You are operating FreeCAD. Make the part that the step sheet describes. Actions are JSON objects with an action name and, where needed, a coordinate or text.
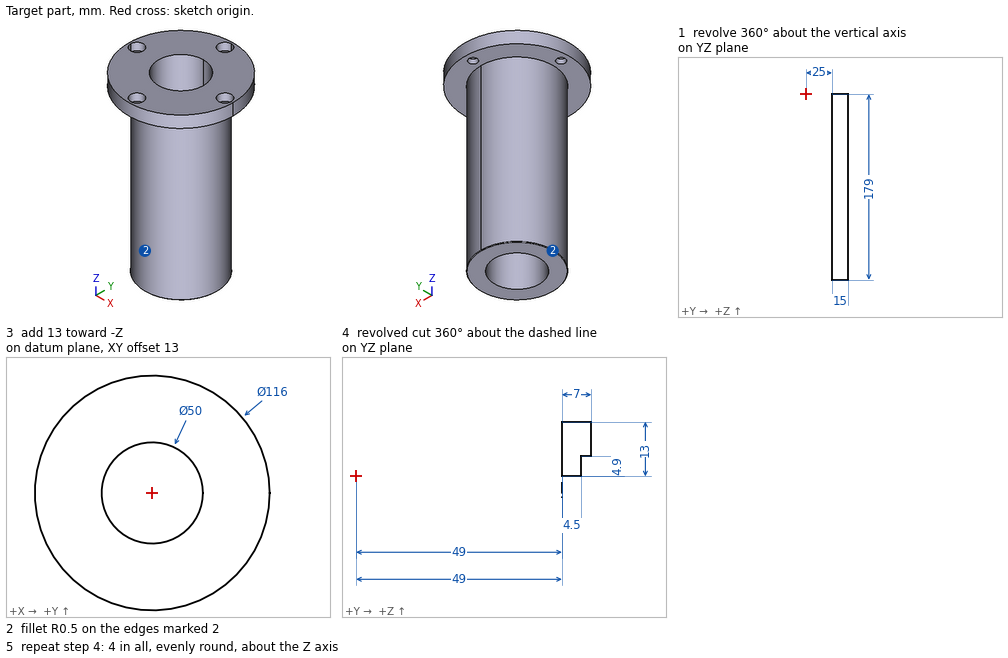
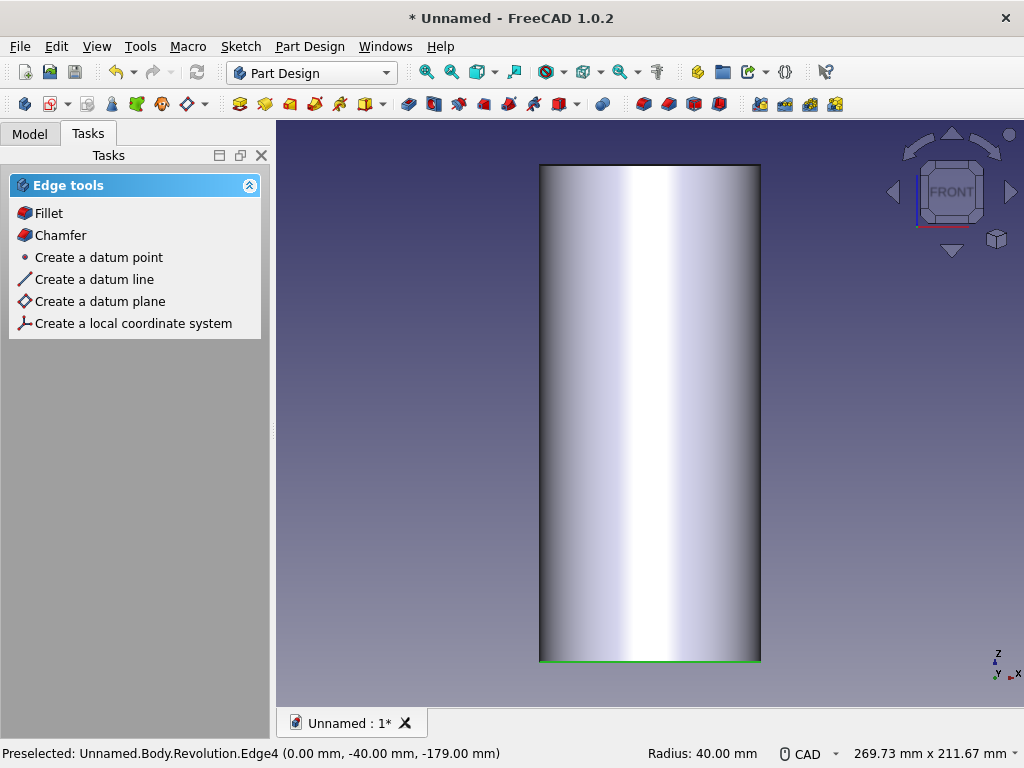
{"action": "left_click", "coordinate": [644, 104]}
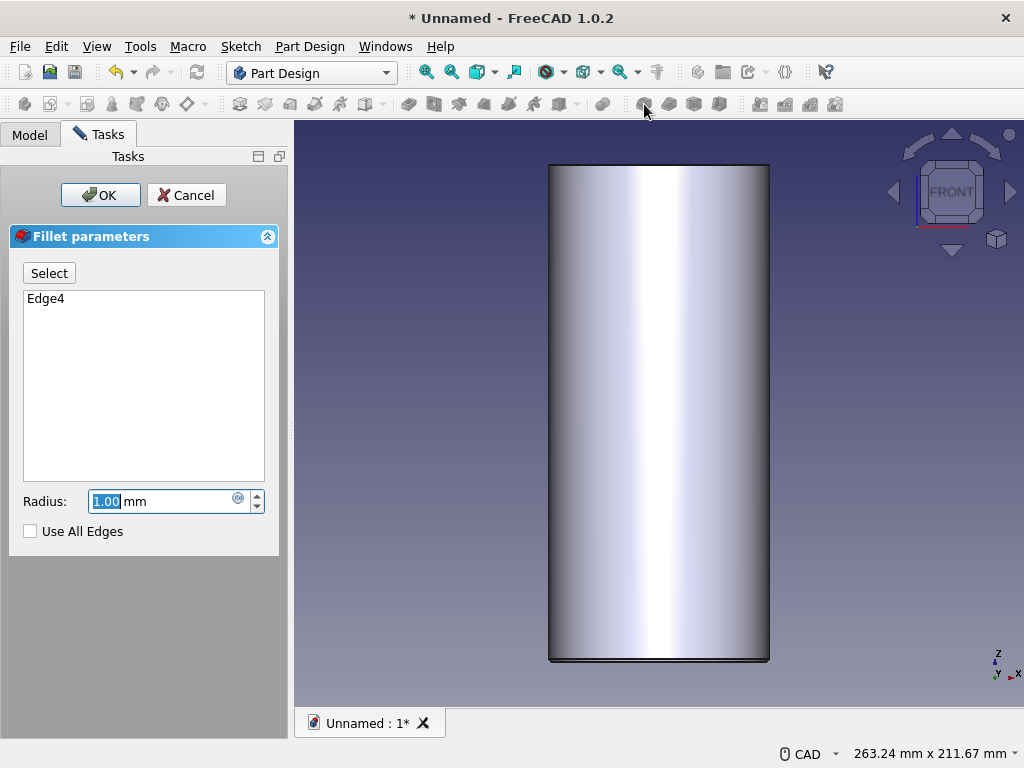
{"action": "type", "text": "0.5"}
{"action": "key", "text": "Tab"}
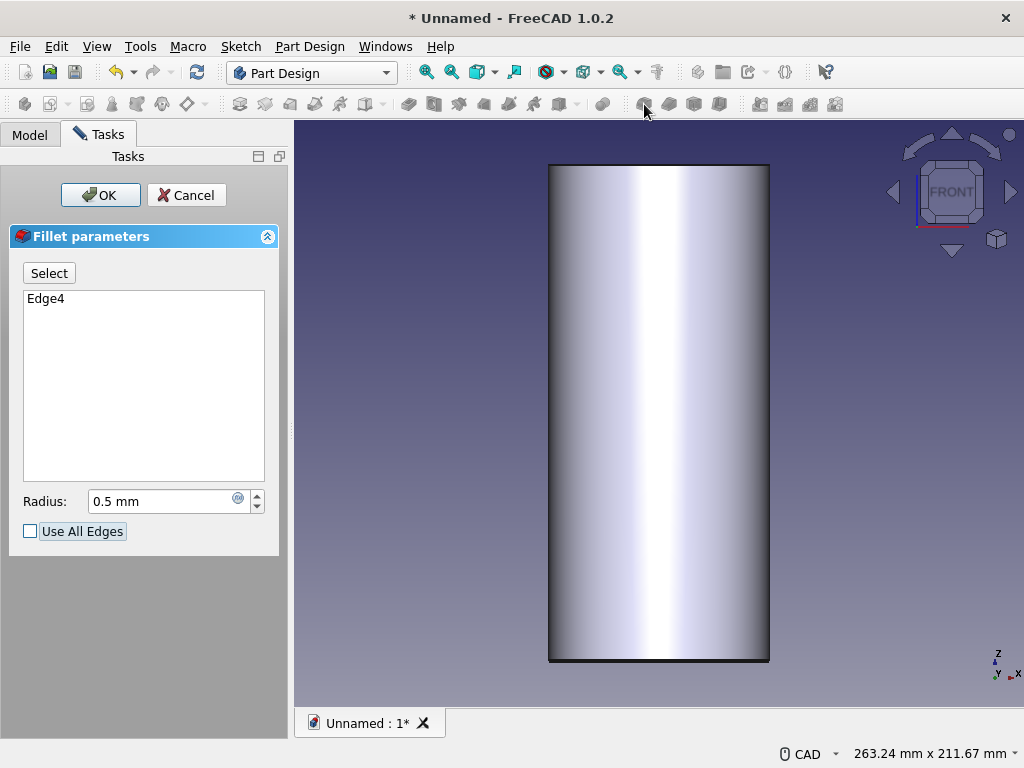
{"action": "left_click", "coordinate": [101, 195]}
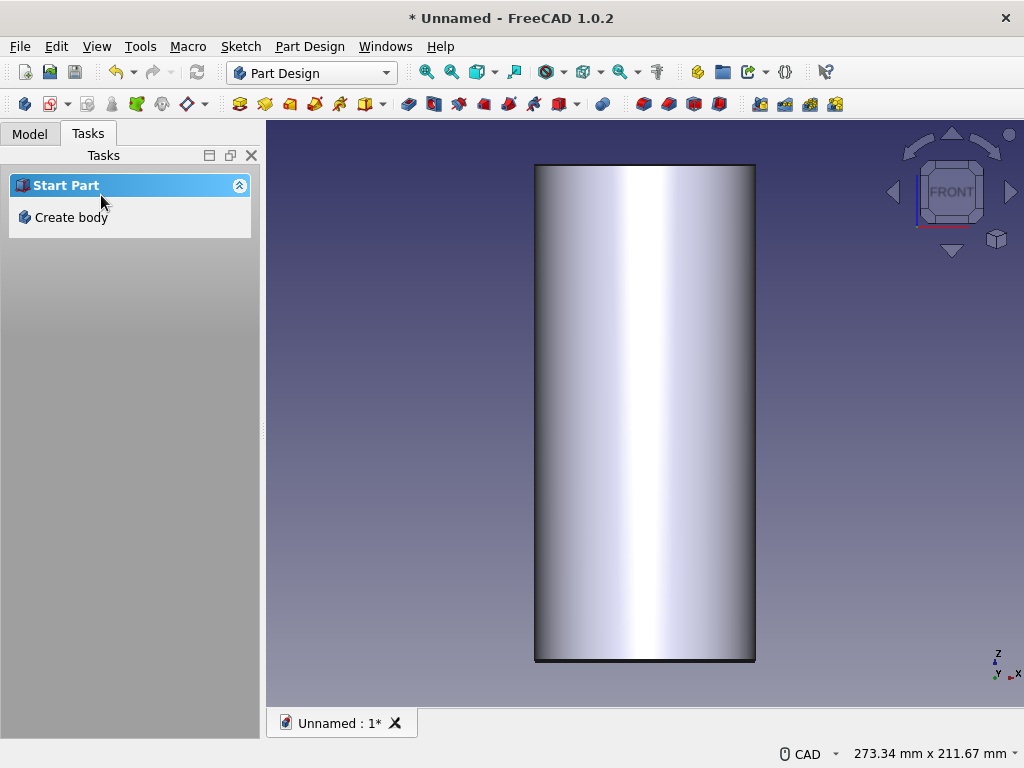
{"action": "left_click", "coordinate": [30, 134]}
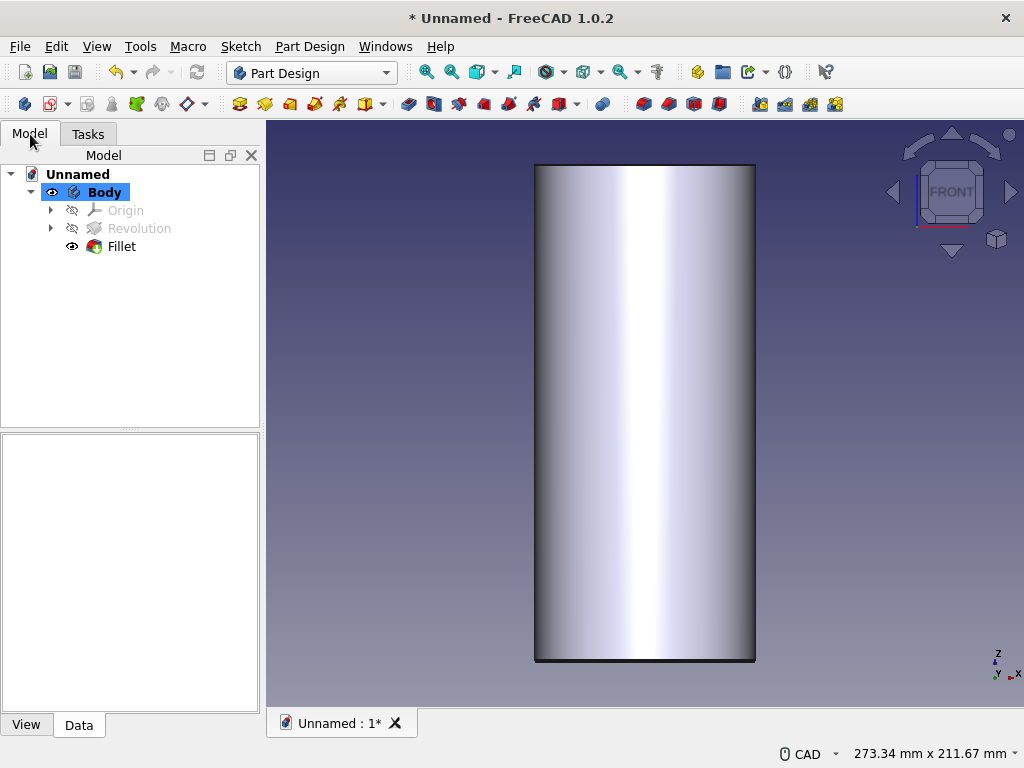
{"action": "left_click", "coordinate": [51, 210]}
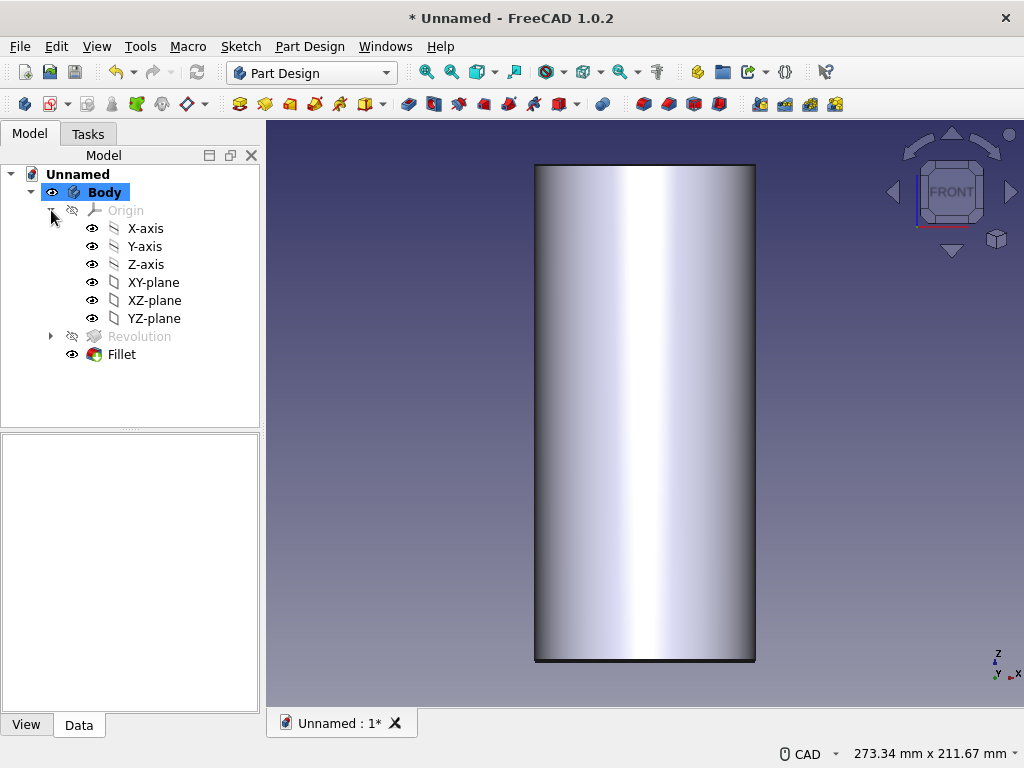
{"action": "left_click", "coordinate": [137, 282]}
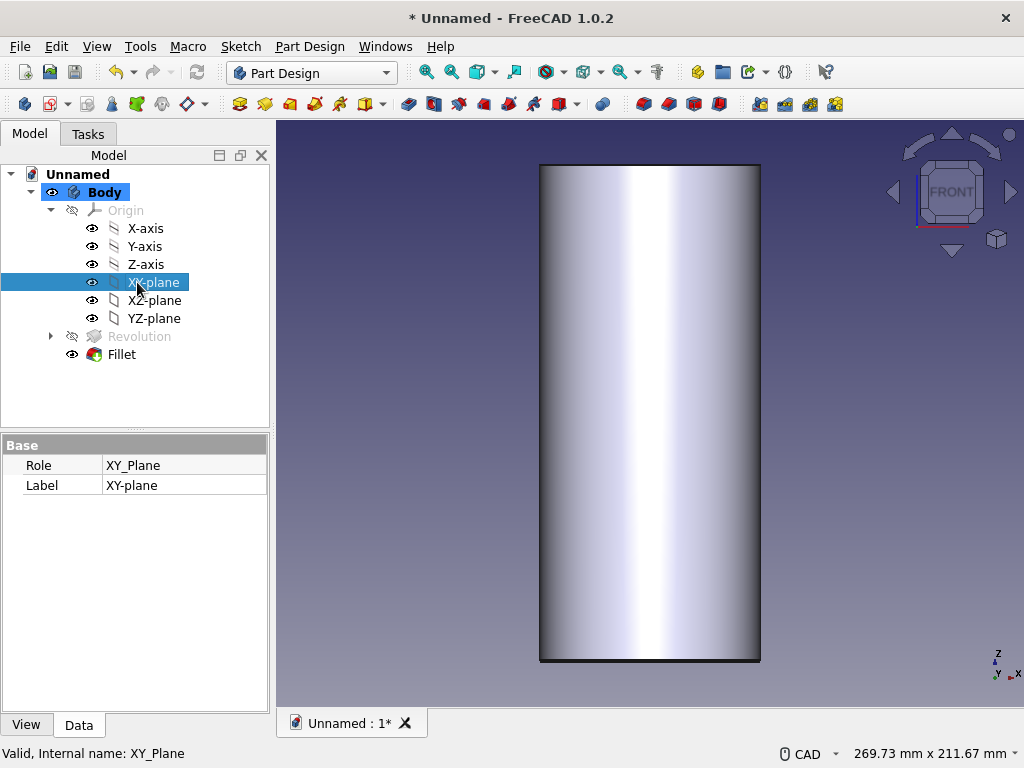
{"action": "left_click", "coordinate": [186, 104]}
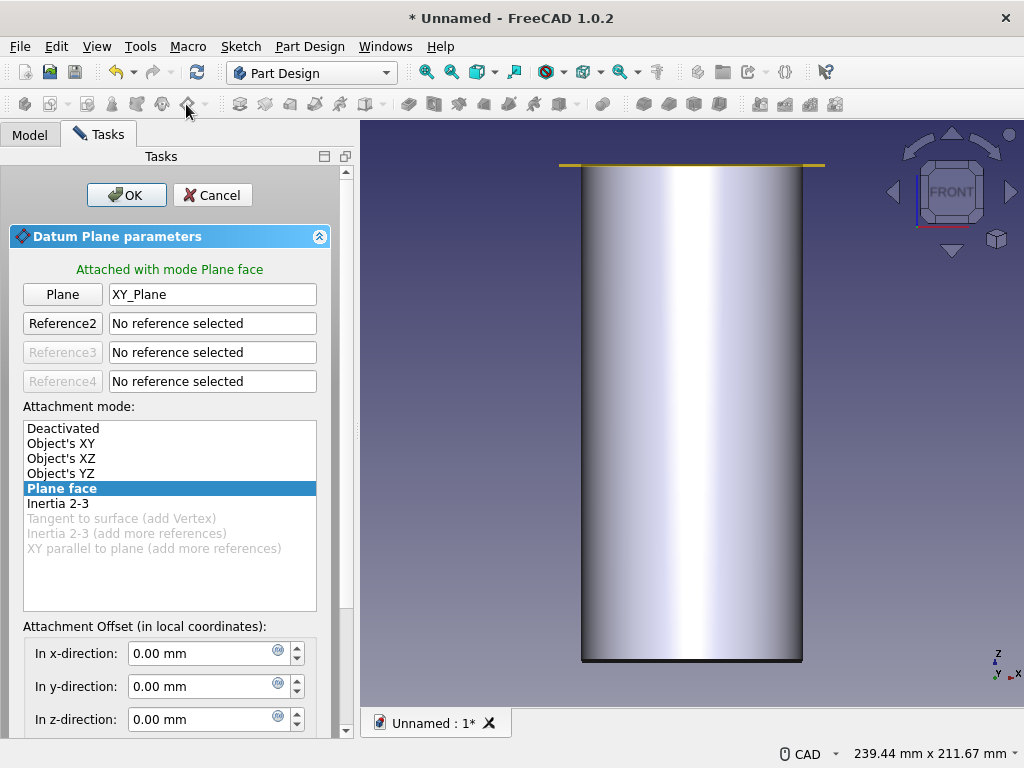
{"action": "triple_click", "coordinate": [210, 720]}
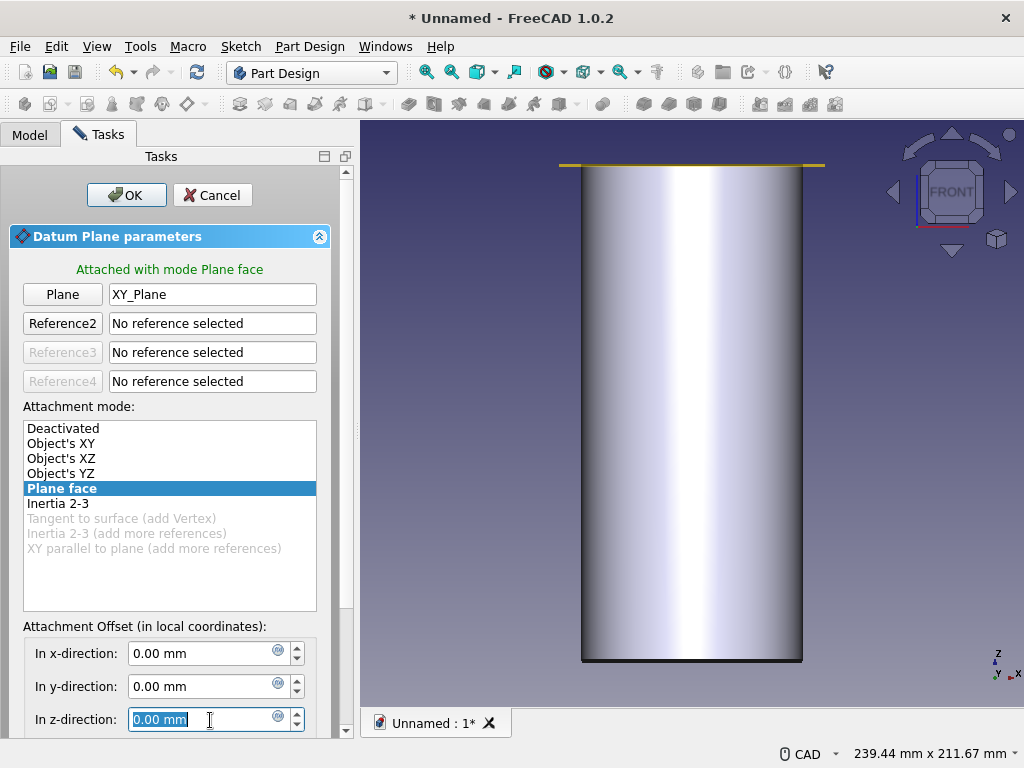
{"action": "type", "text": "13"}
{"action": "key", "text": "Tab"}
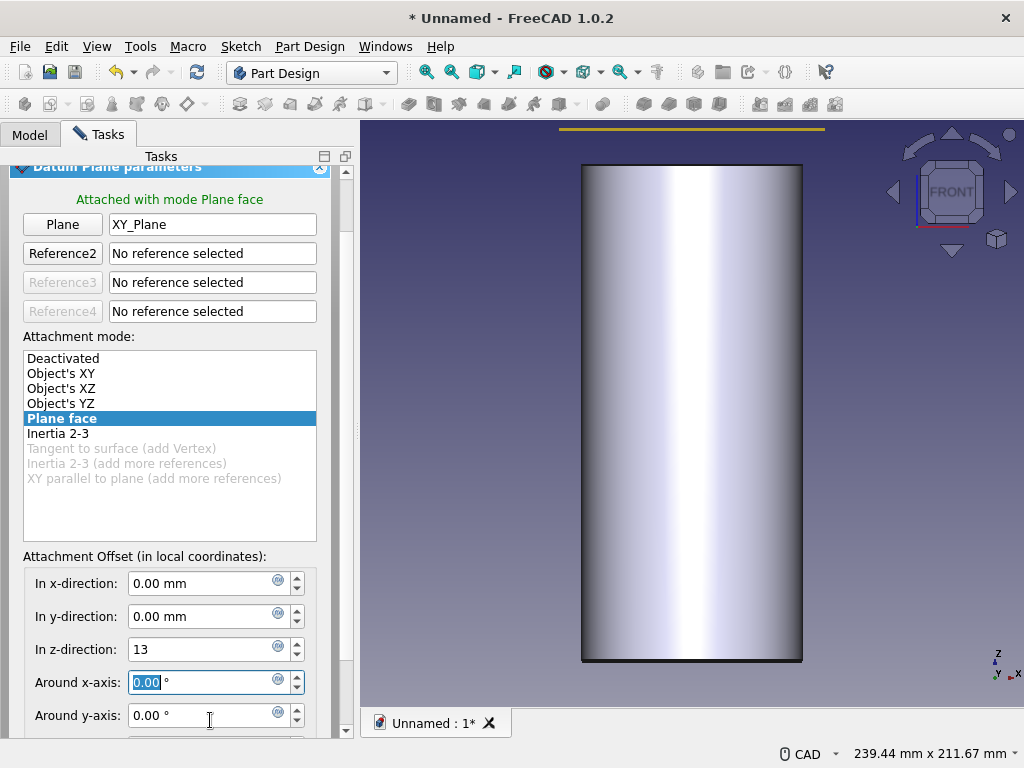
{"action": "scroll", "coordinate": [346, 452], "scroll_direction": "up", "scroll_amount": 2}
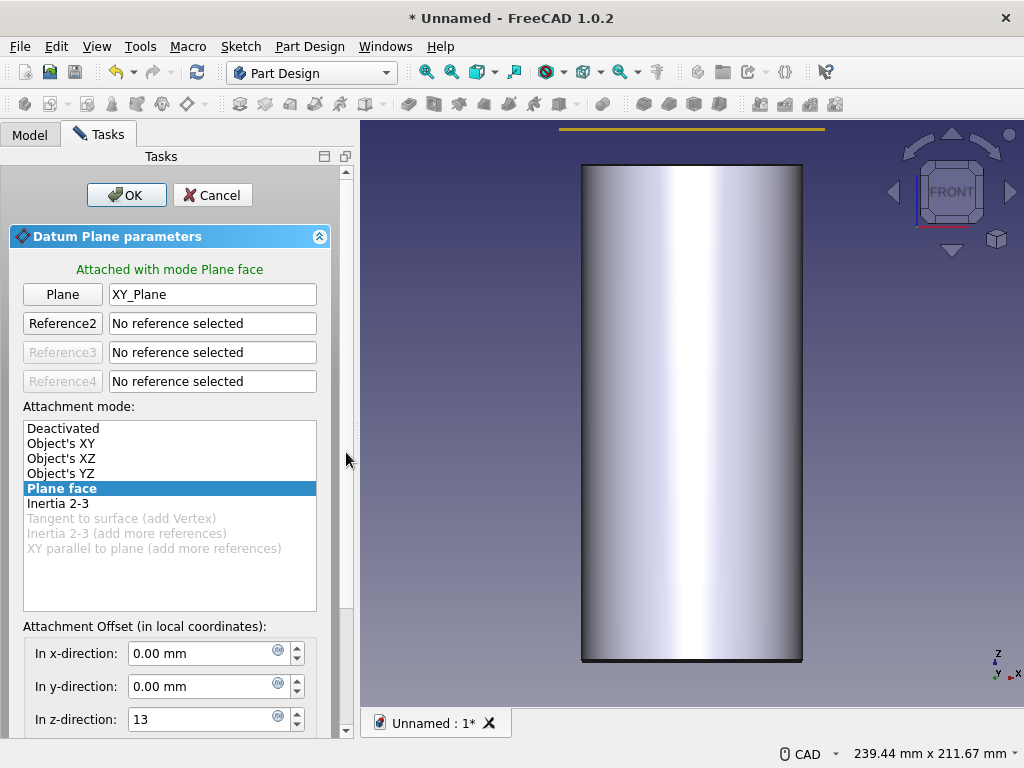
{"action": "left_click", "coordinate": [127, 195]}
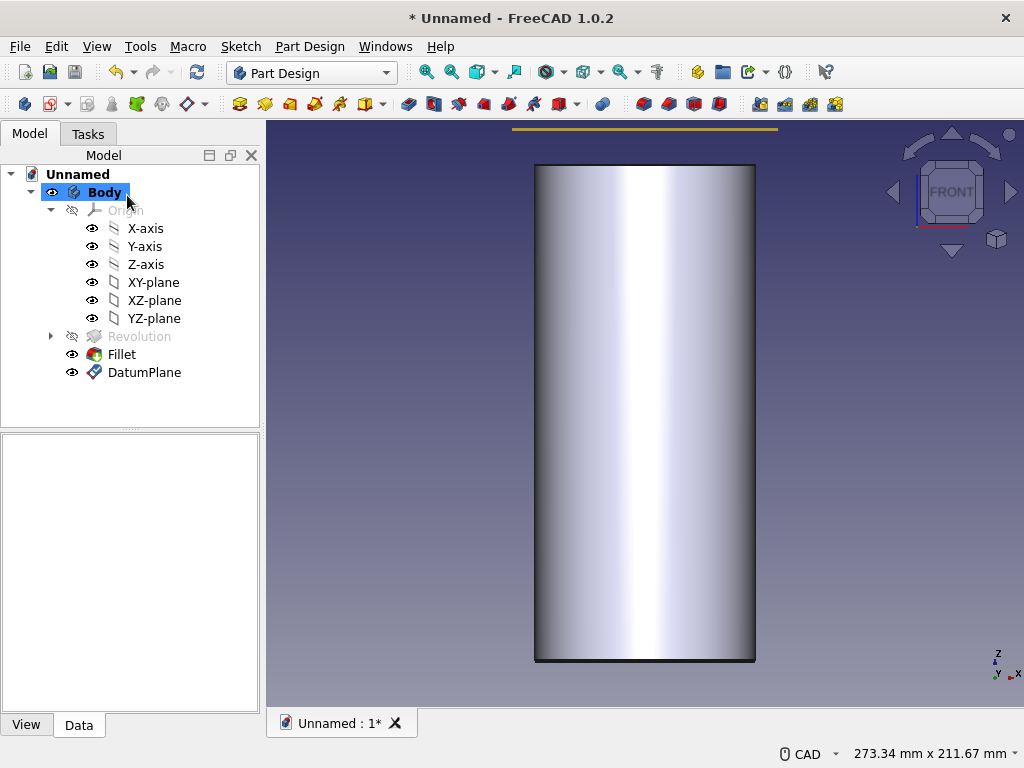
{"action": "left_click", "coordinate": [117, 372]}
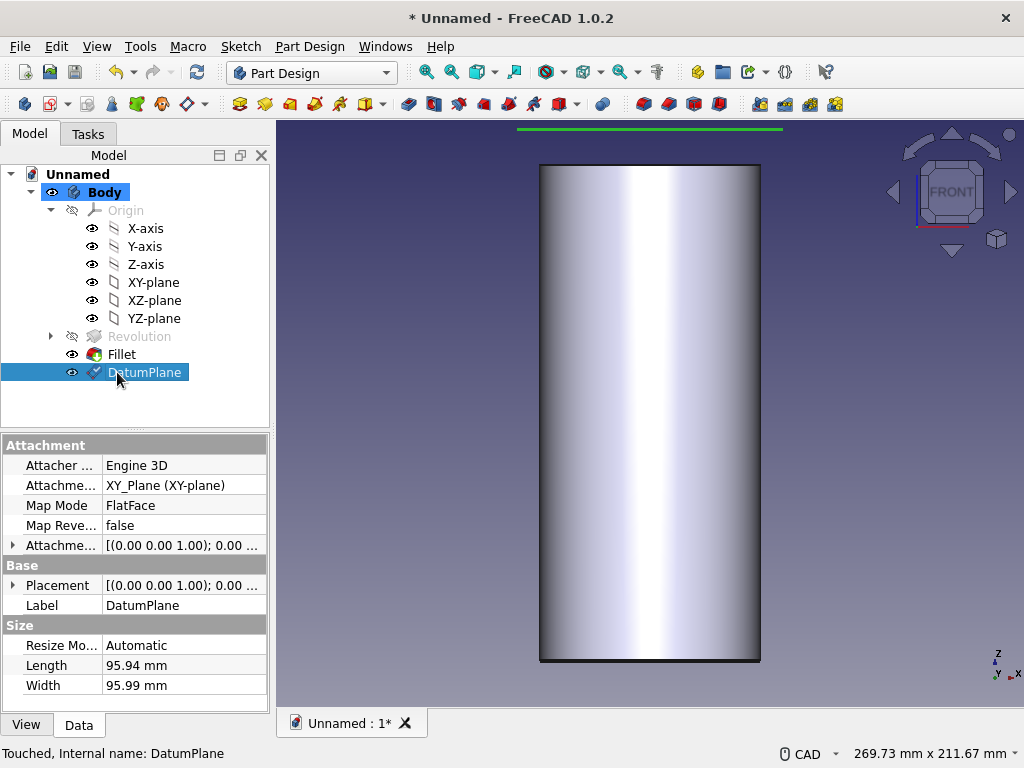
{"action": "left_click", "coordinate": [50, 104]}